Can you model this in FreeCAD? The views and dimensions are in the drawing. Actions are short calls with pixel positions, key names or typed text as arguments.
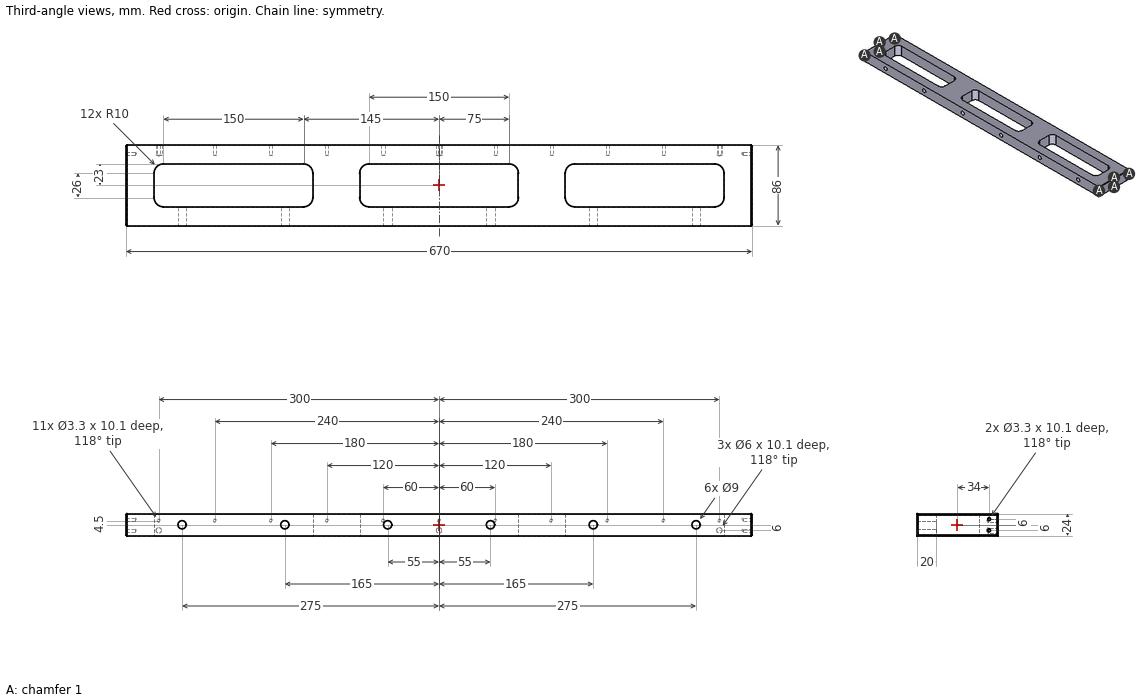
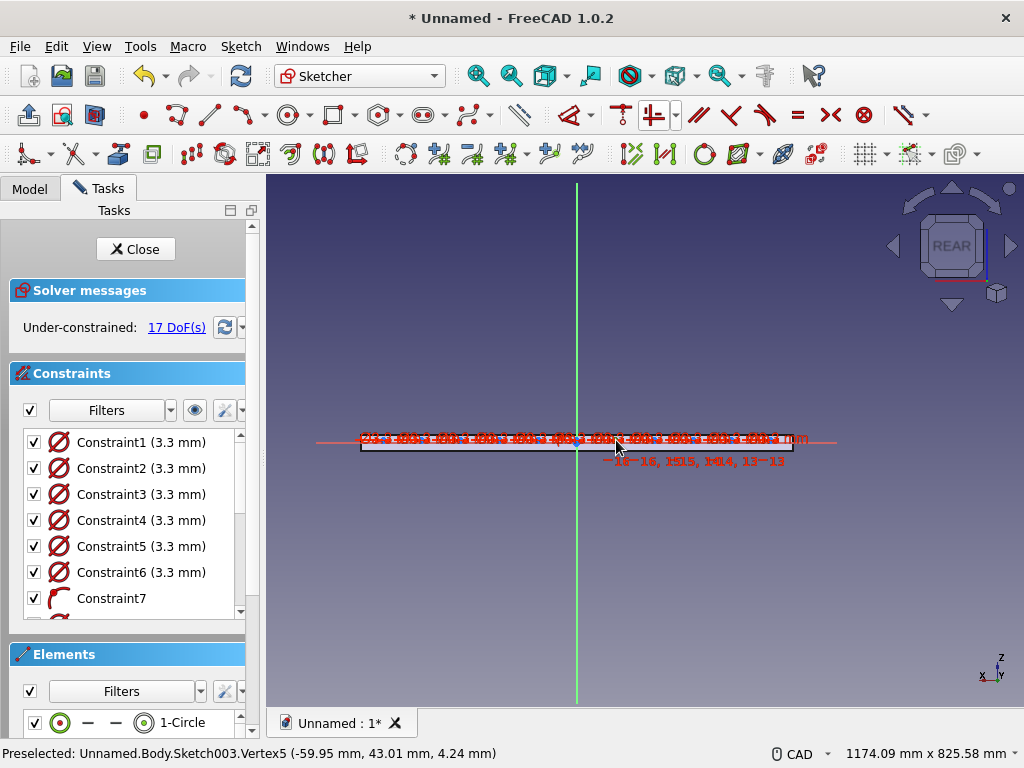
scroll(577, 440, up, 8)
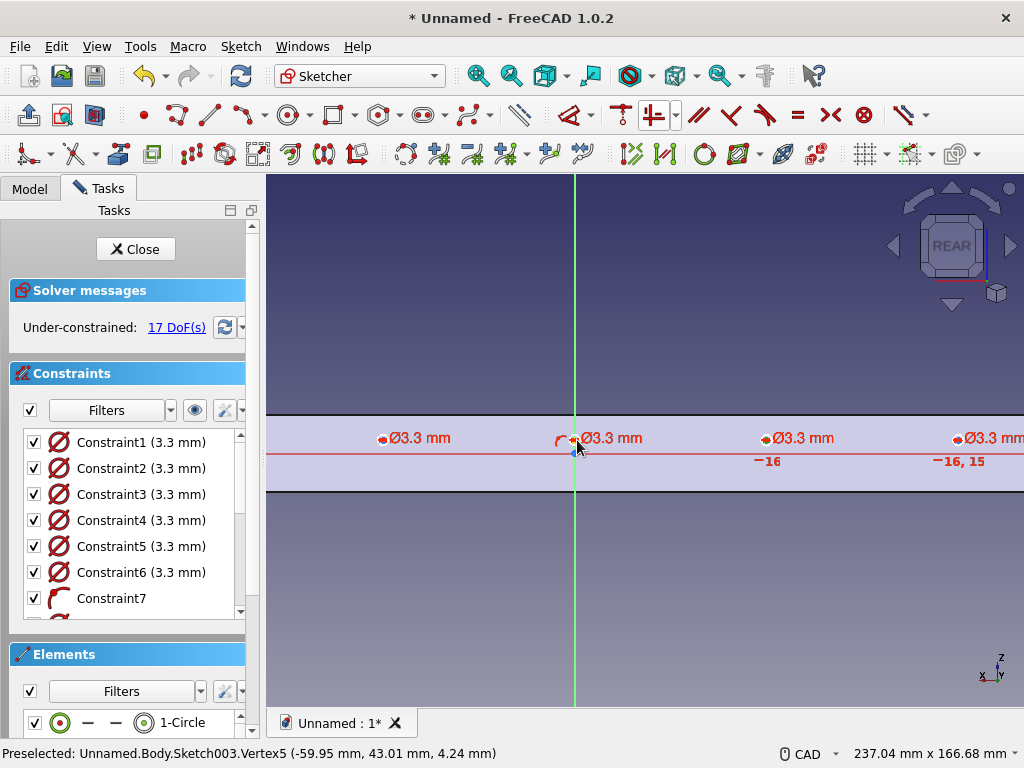
click(575, 440)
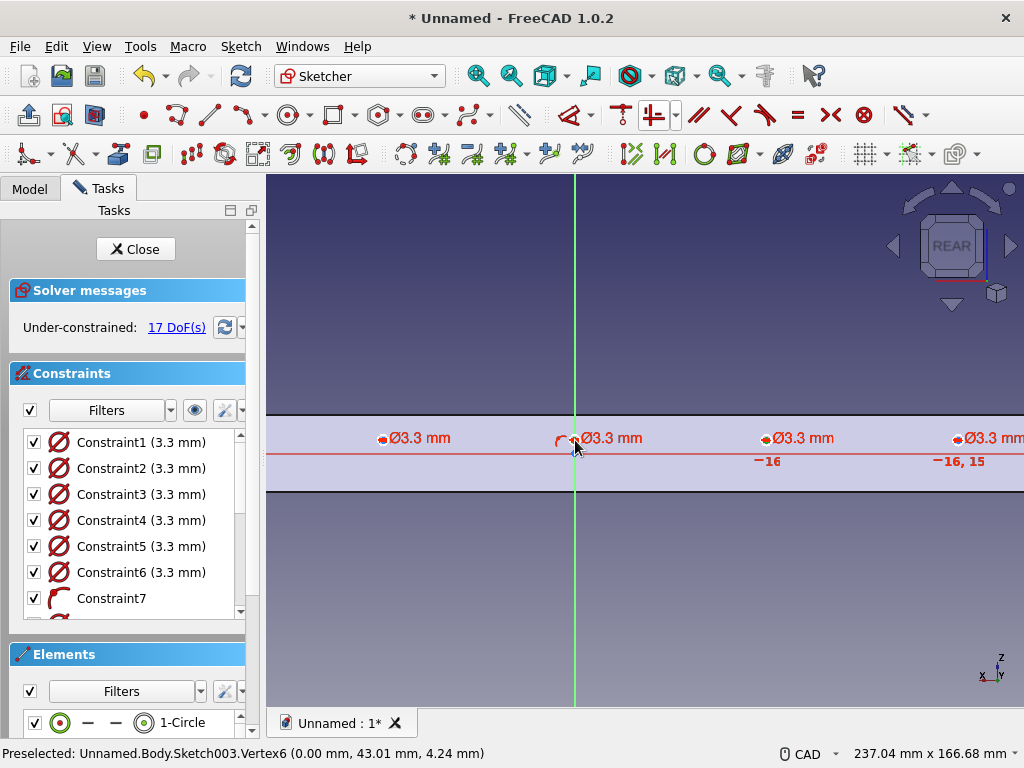
key(h)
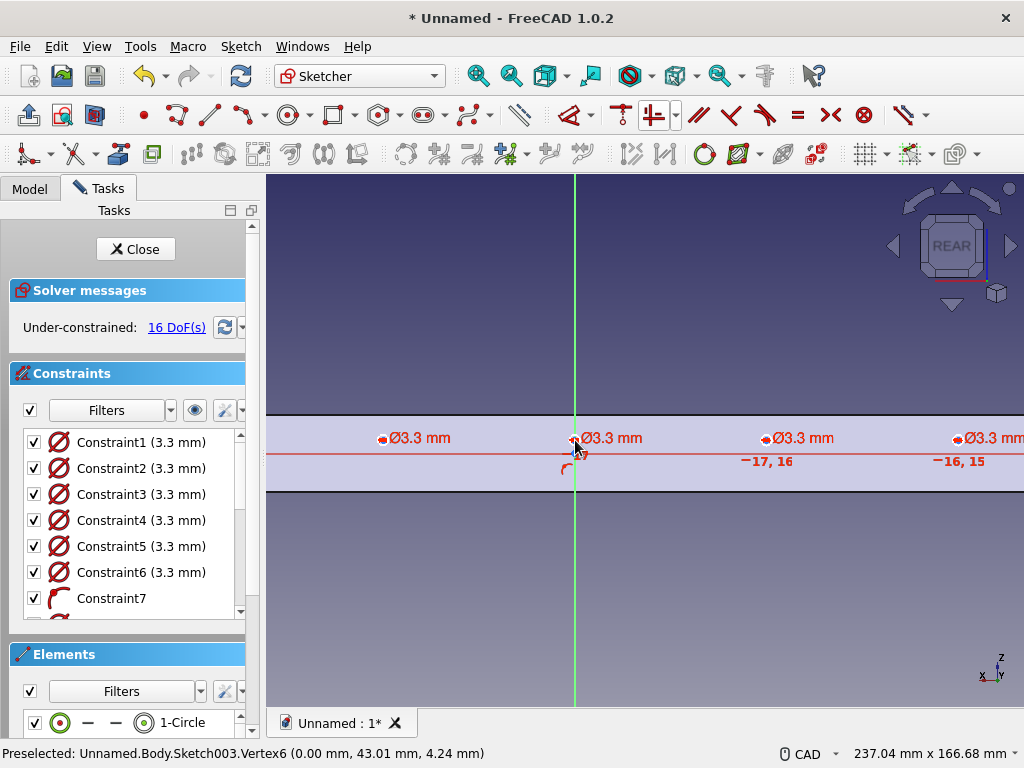
click(575, 440)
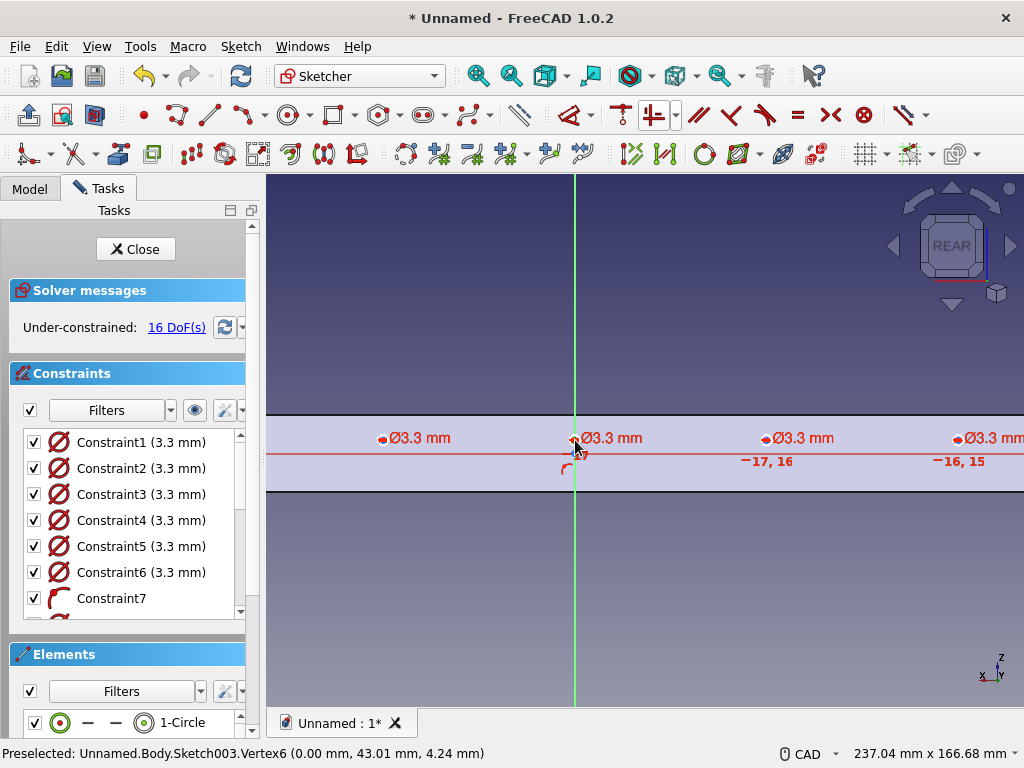
scroll(577, 440, down, 8)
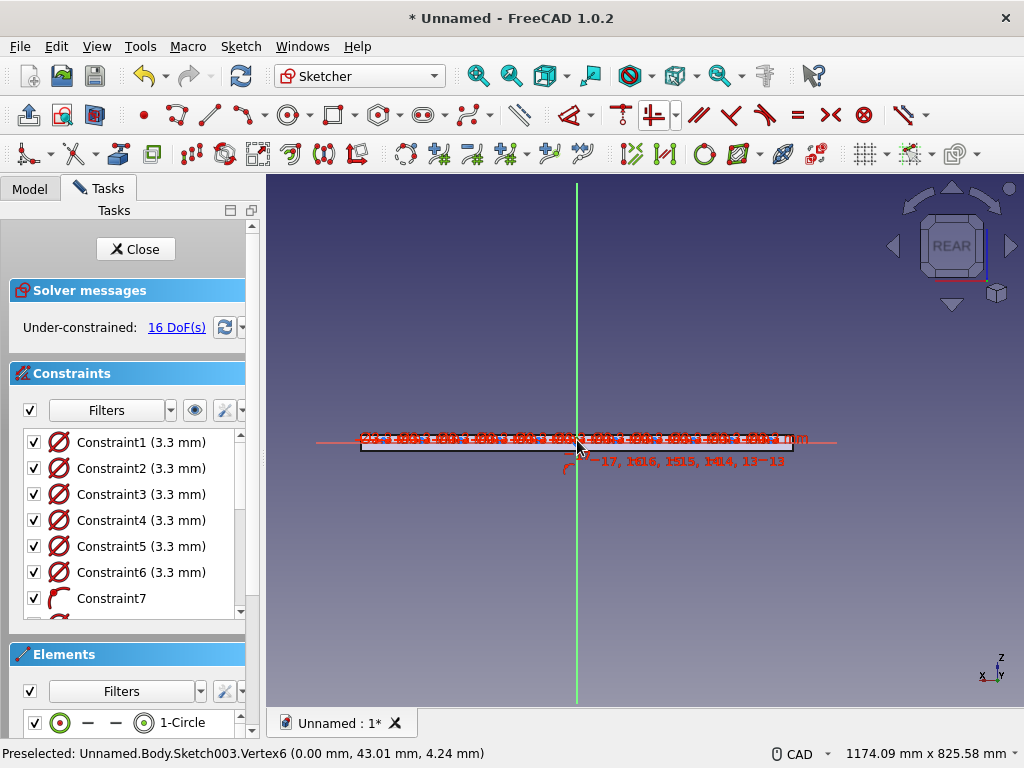
click(538, 440)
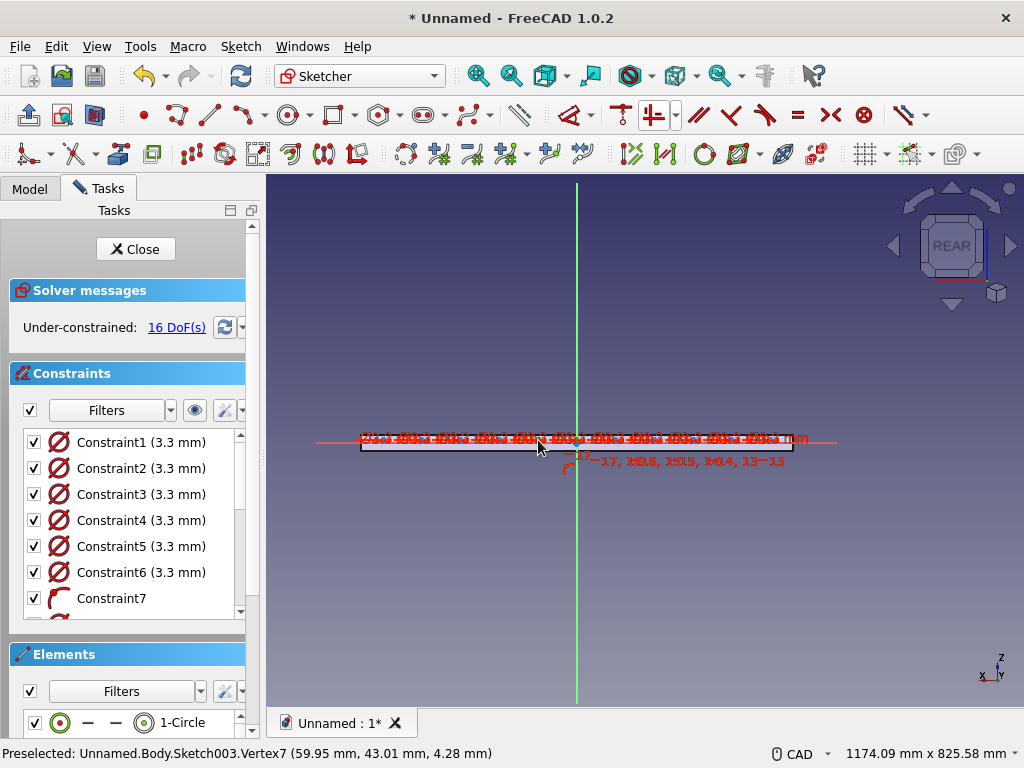
key(h)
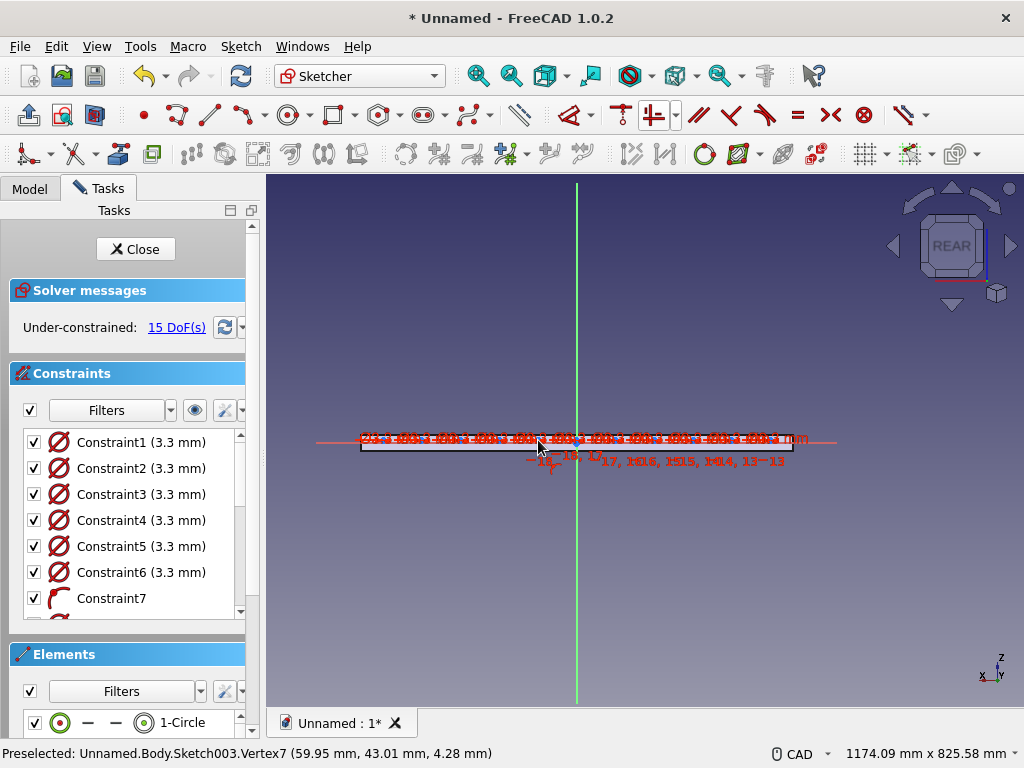
click(538, 440)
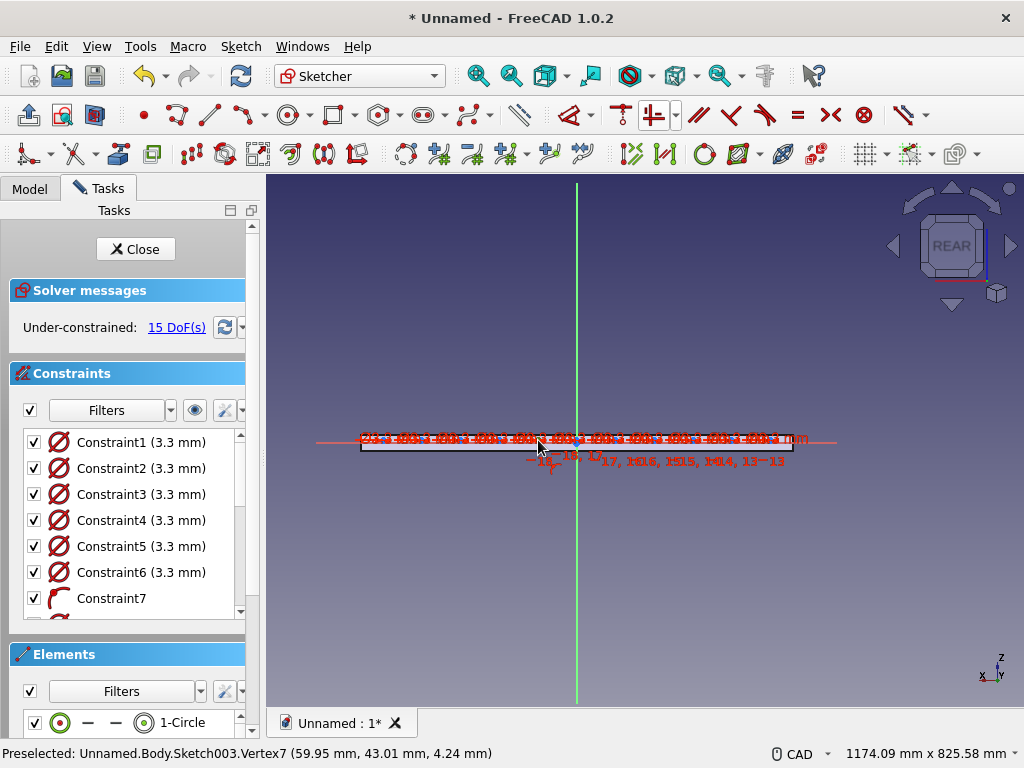
click(499, 440)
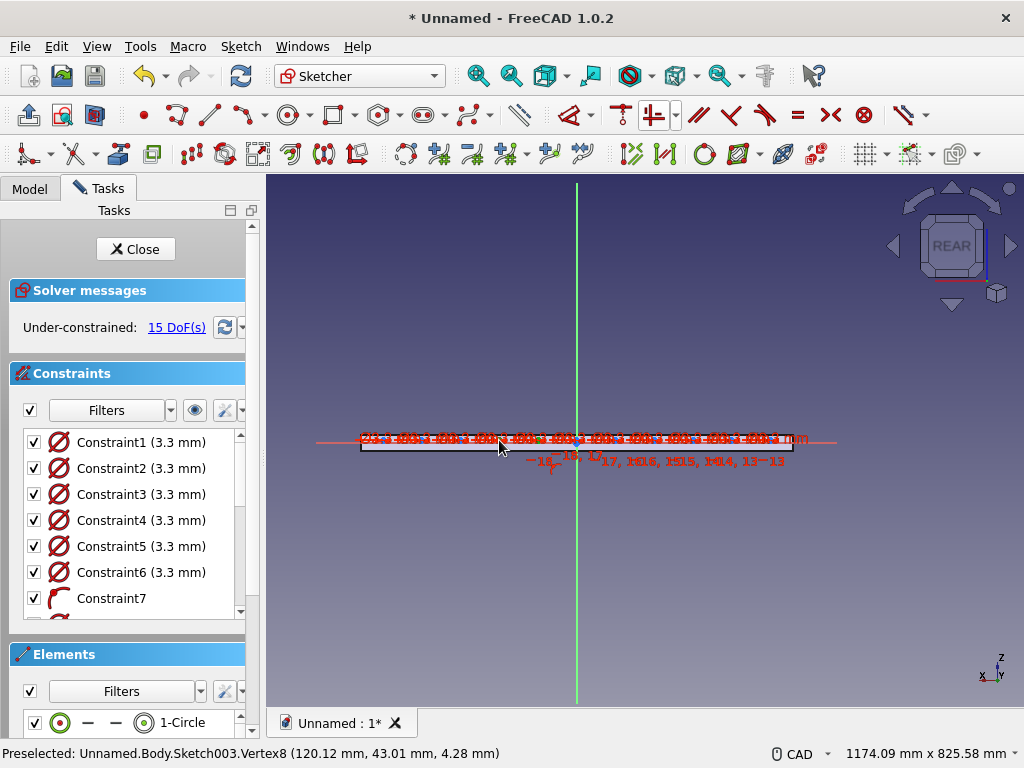
key(h)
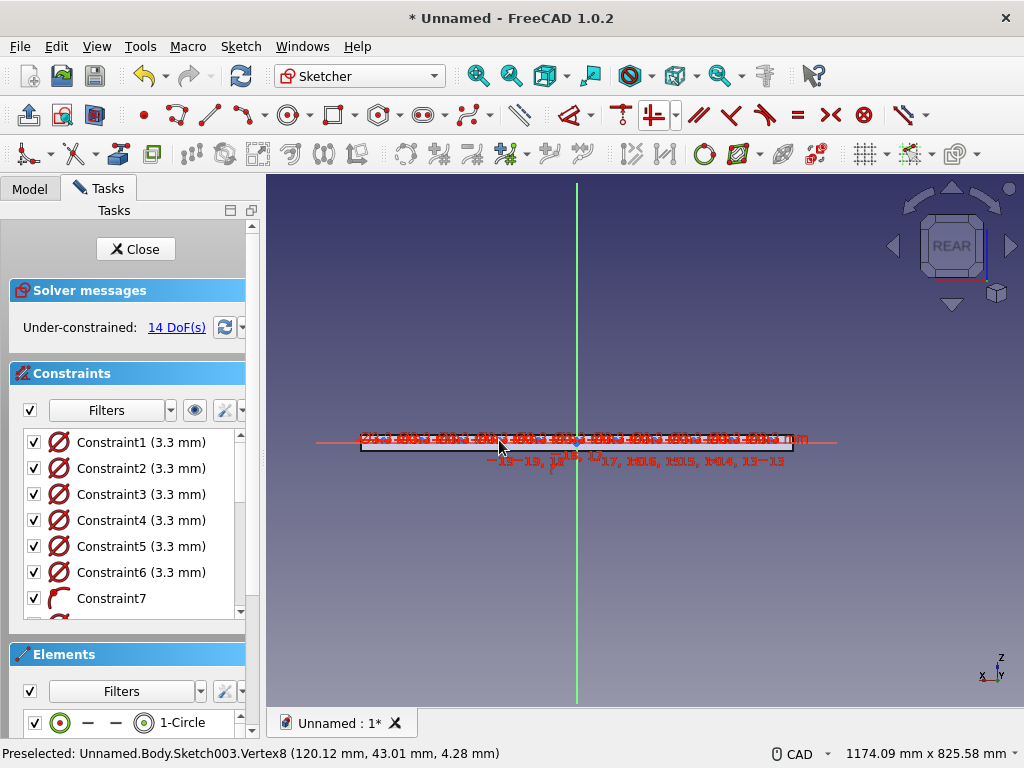
click(499, 440)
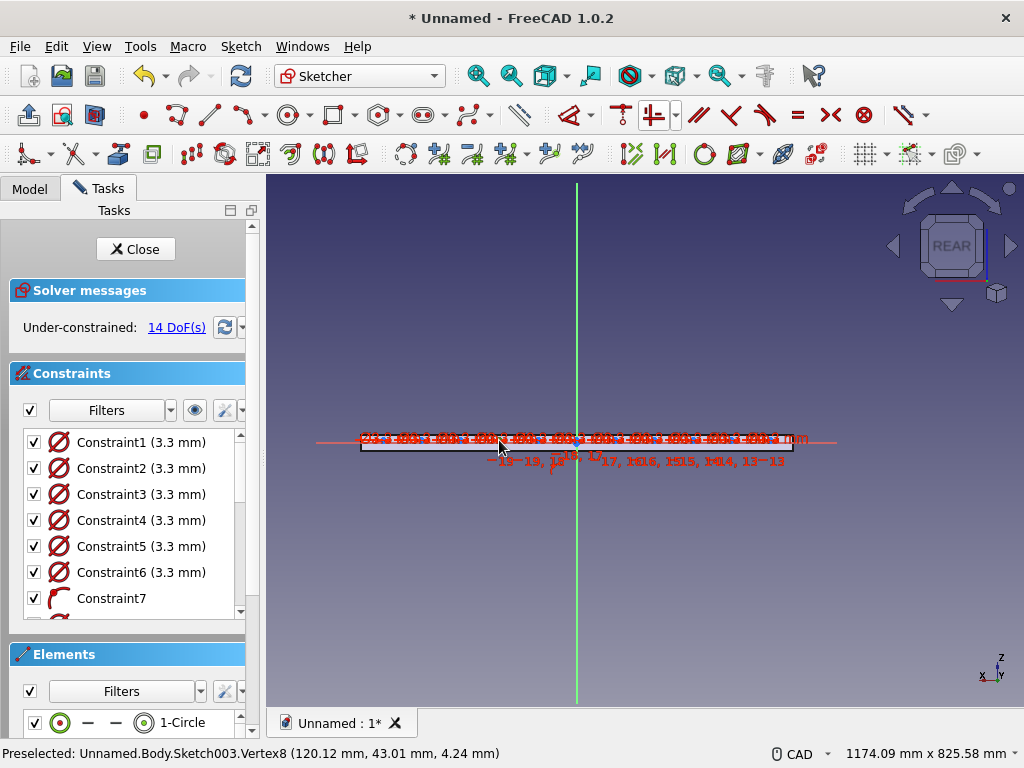
click(461, 440)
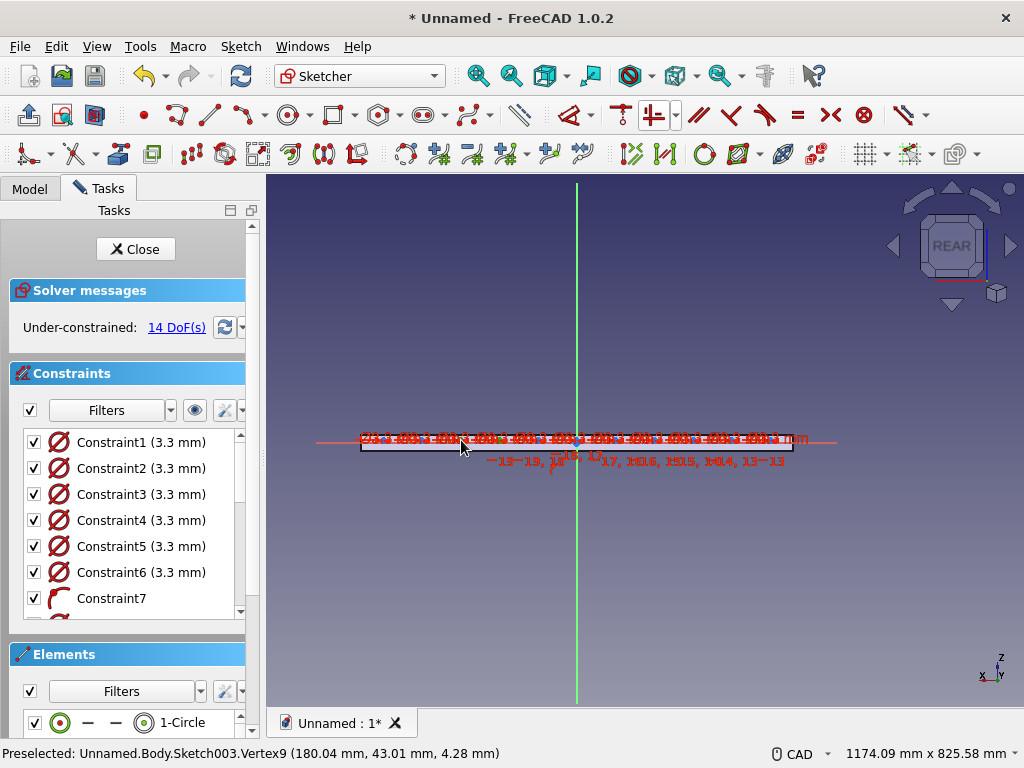
key(h)